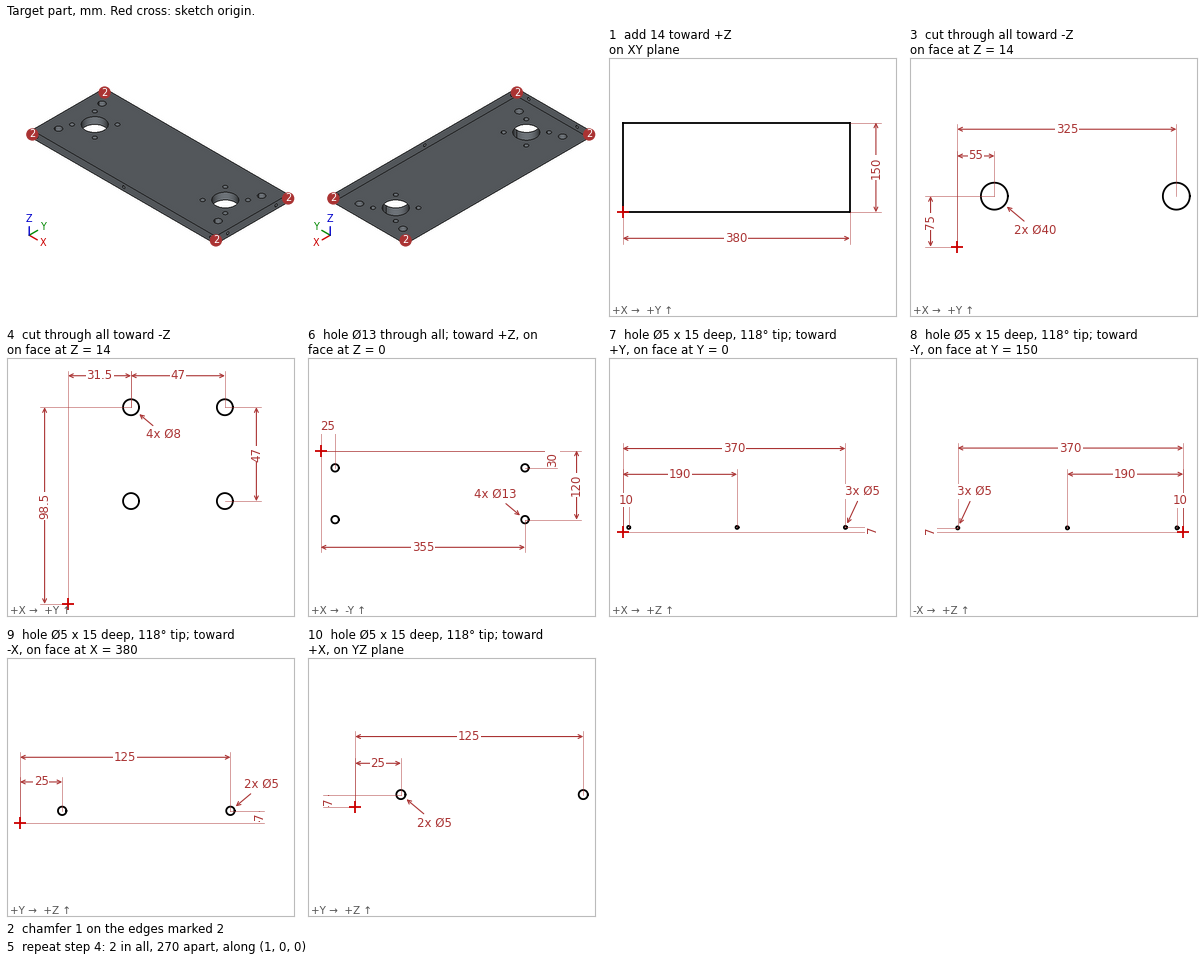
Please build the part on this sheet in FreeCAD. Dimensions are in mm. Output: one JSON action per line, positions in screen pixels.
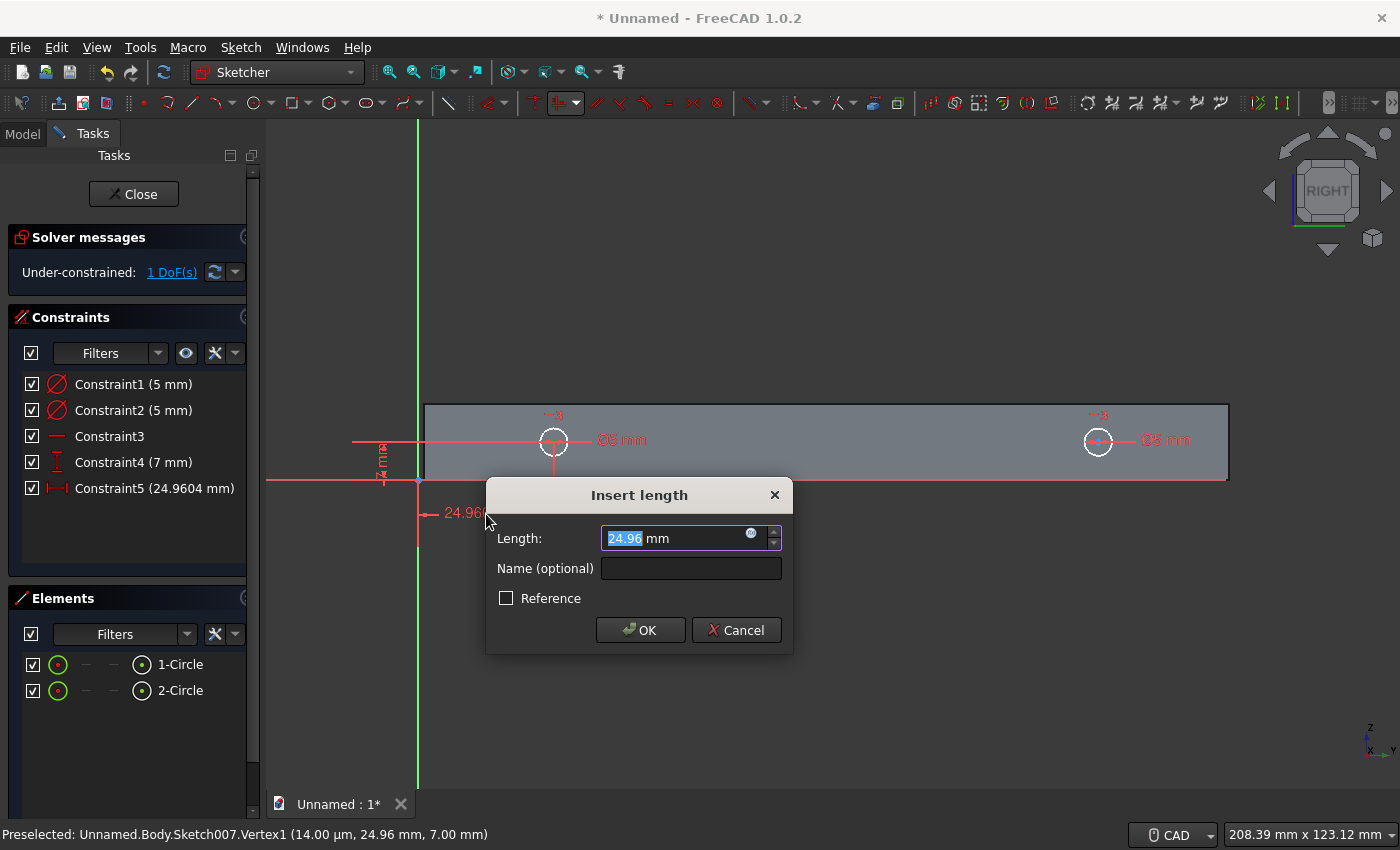
{"action": "type", "text": "25"}
{"action": "key", "text": "Return"}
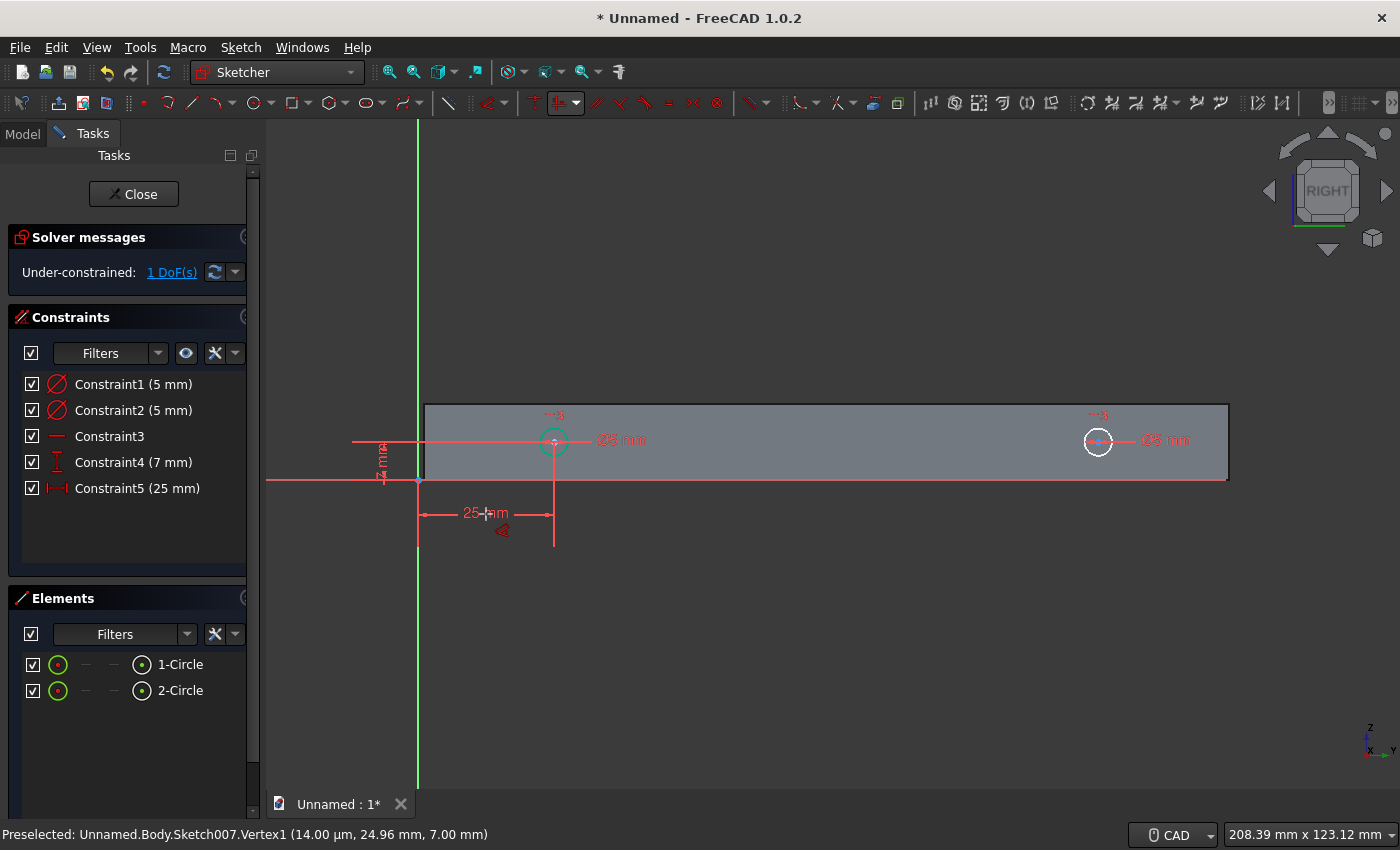
{"action": "left_click", "coordinate": [1098, 442]}
{"action": "left_click", "coordinate": [758, 514]}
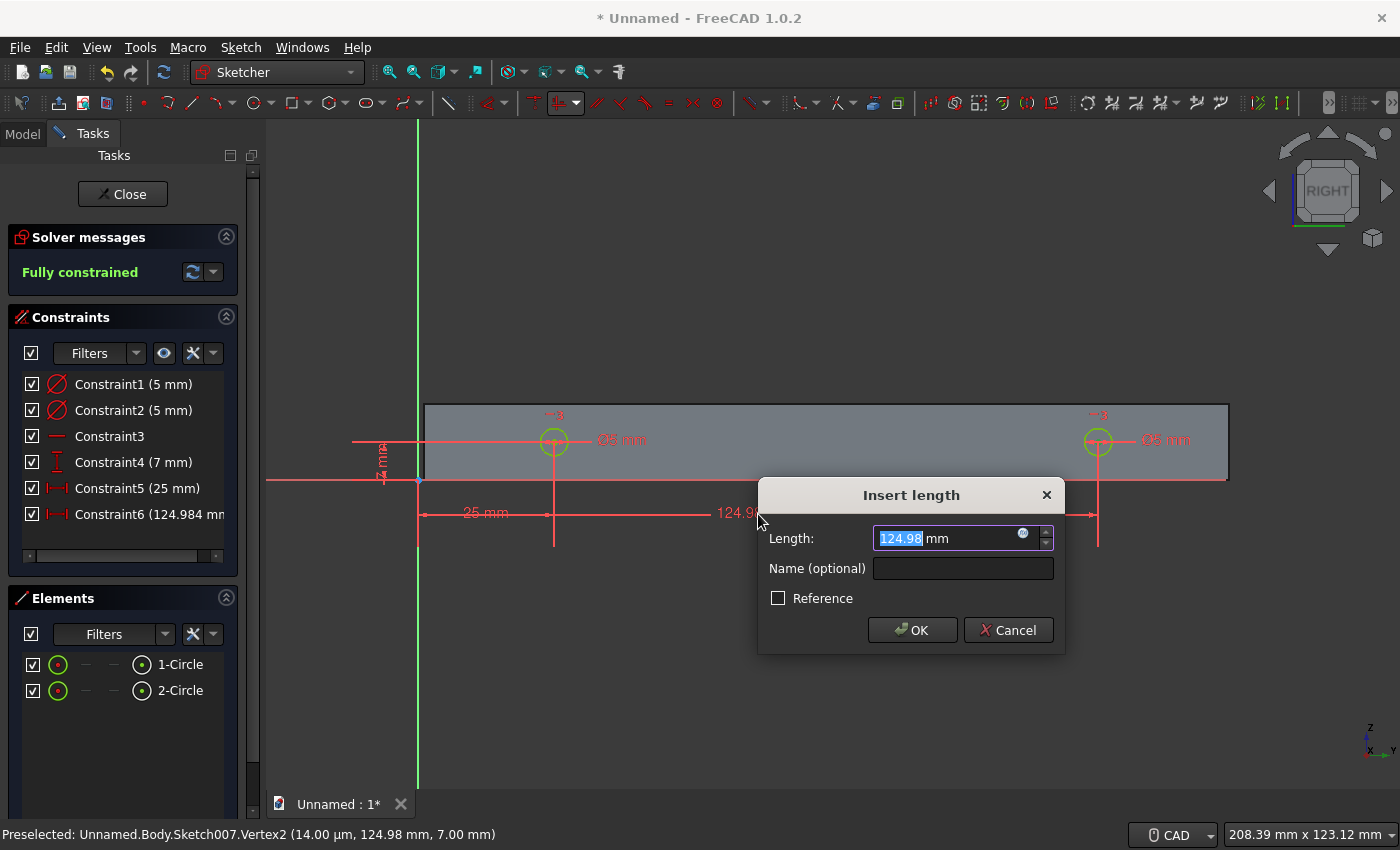
{"action": "type", "text": "125"}
{"action": "key", "text": "Return"}
{"action": "key", "text": "Escape"}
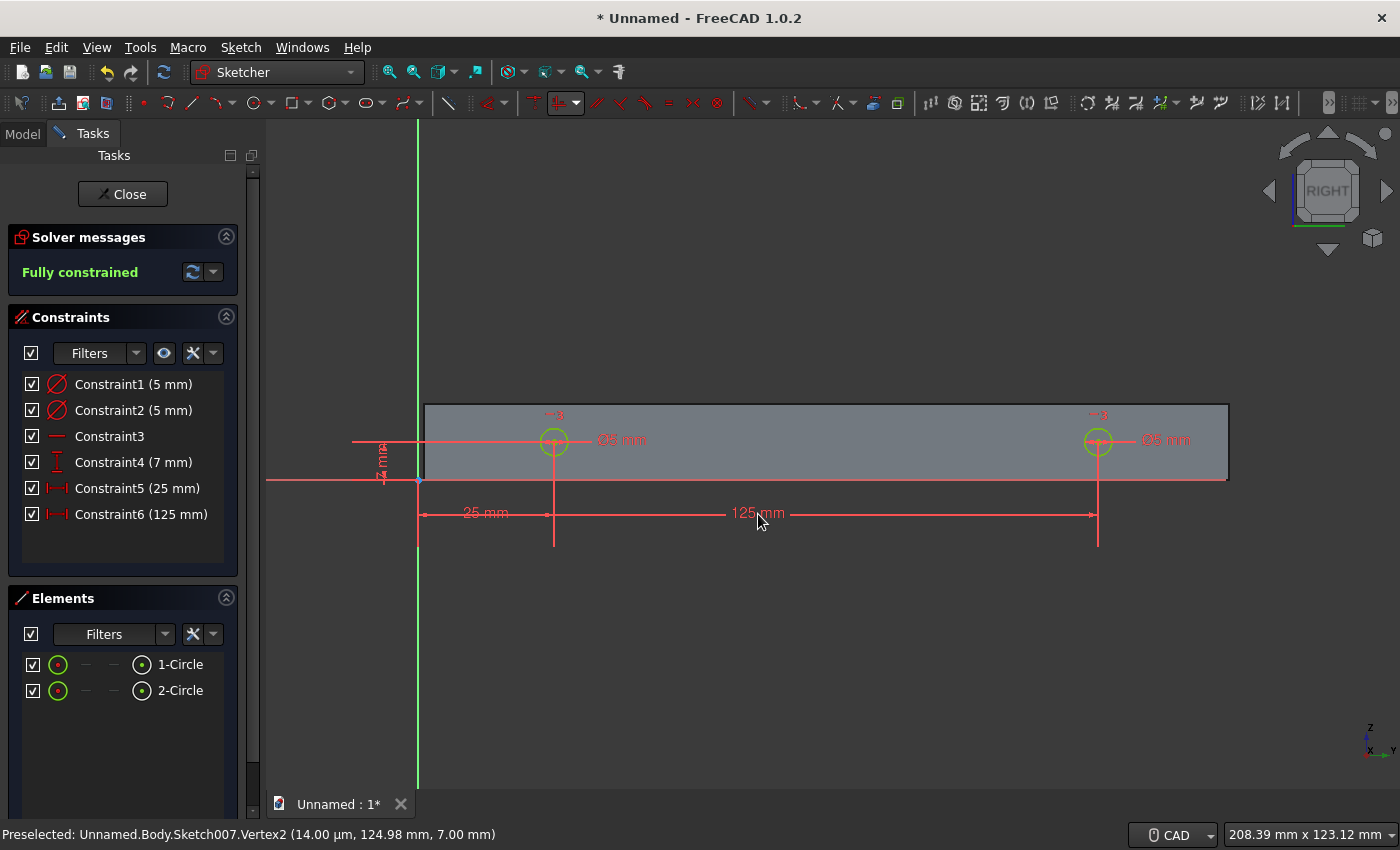
{"action": "left_click", "coordinate": [123, 194]}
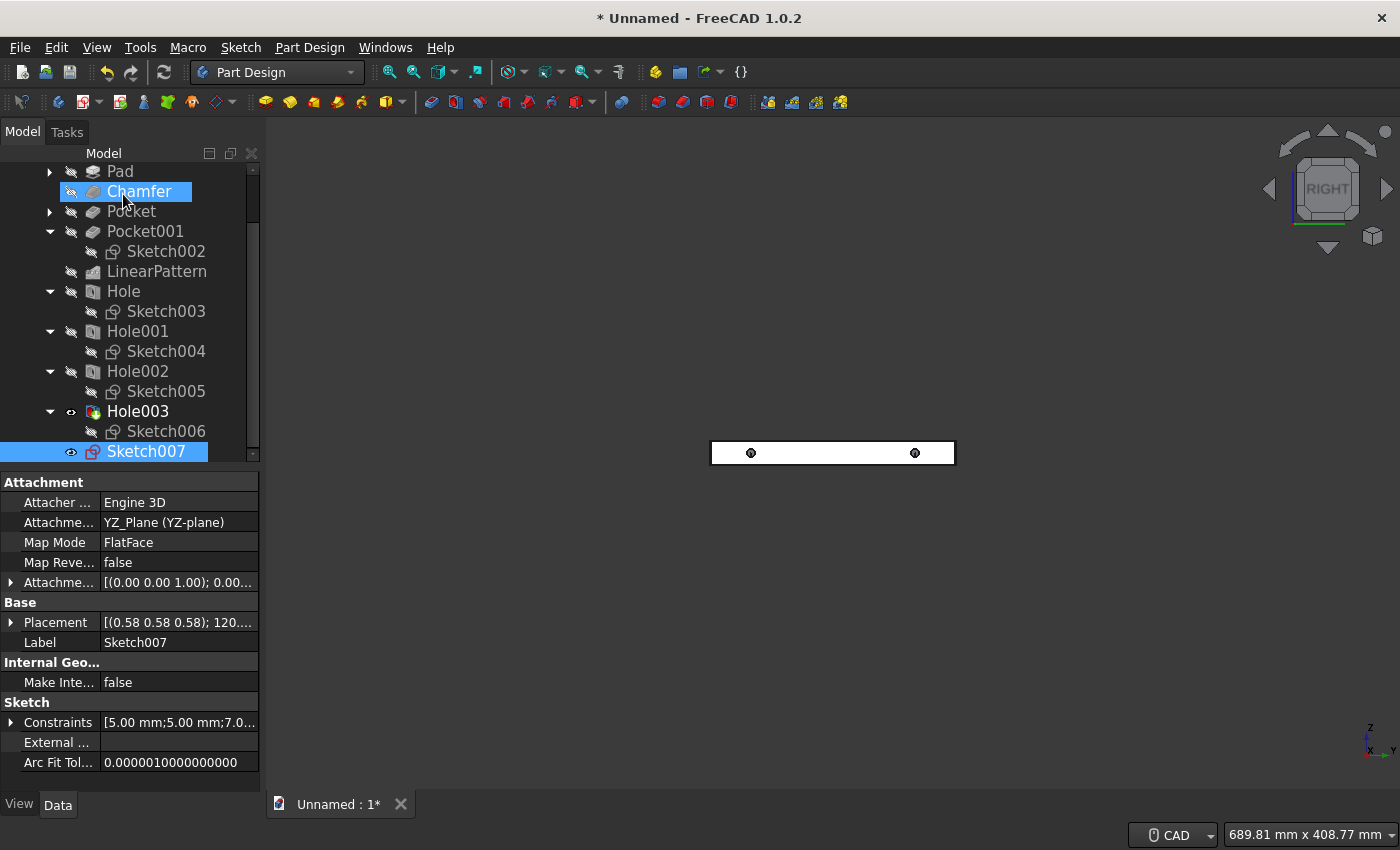
{"action": "left_click", "coordinate": [456, 102]}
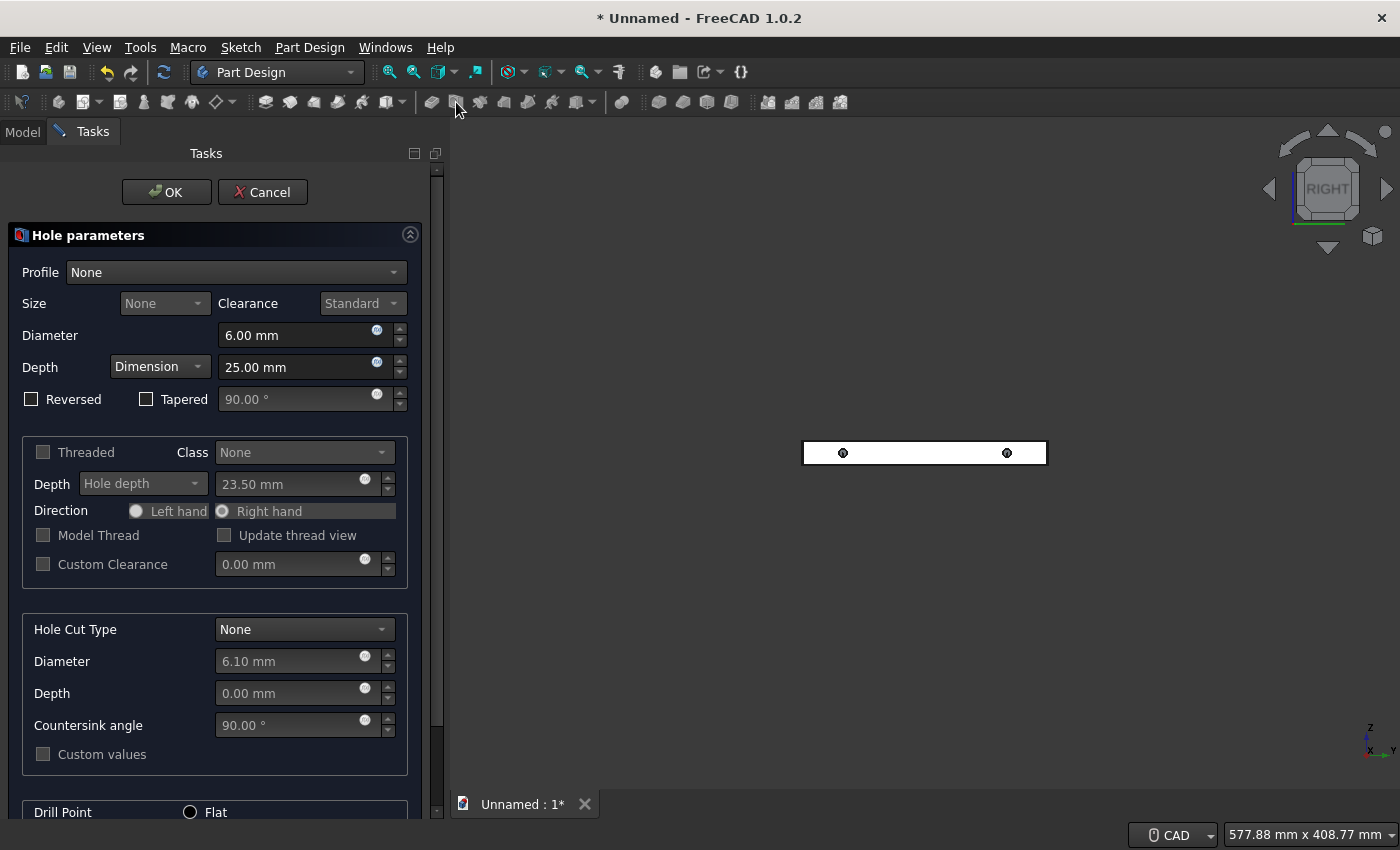
{"action": "triple_click", "coordinate": [305, 335]}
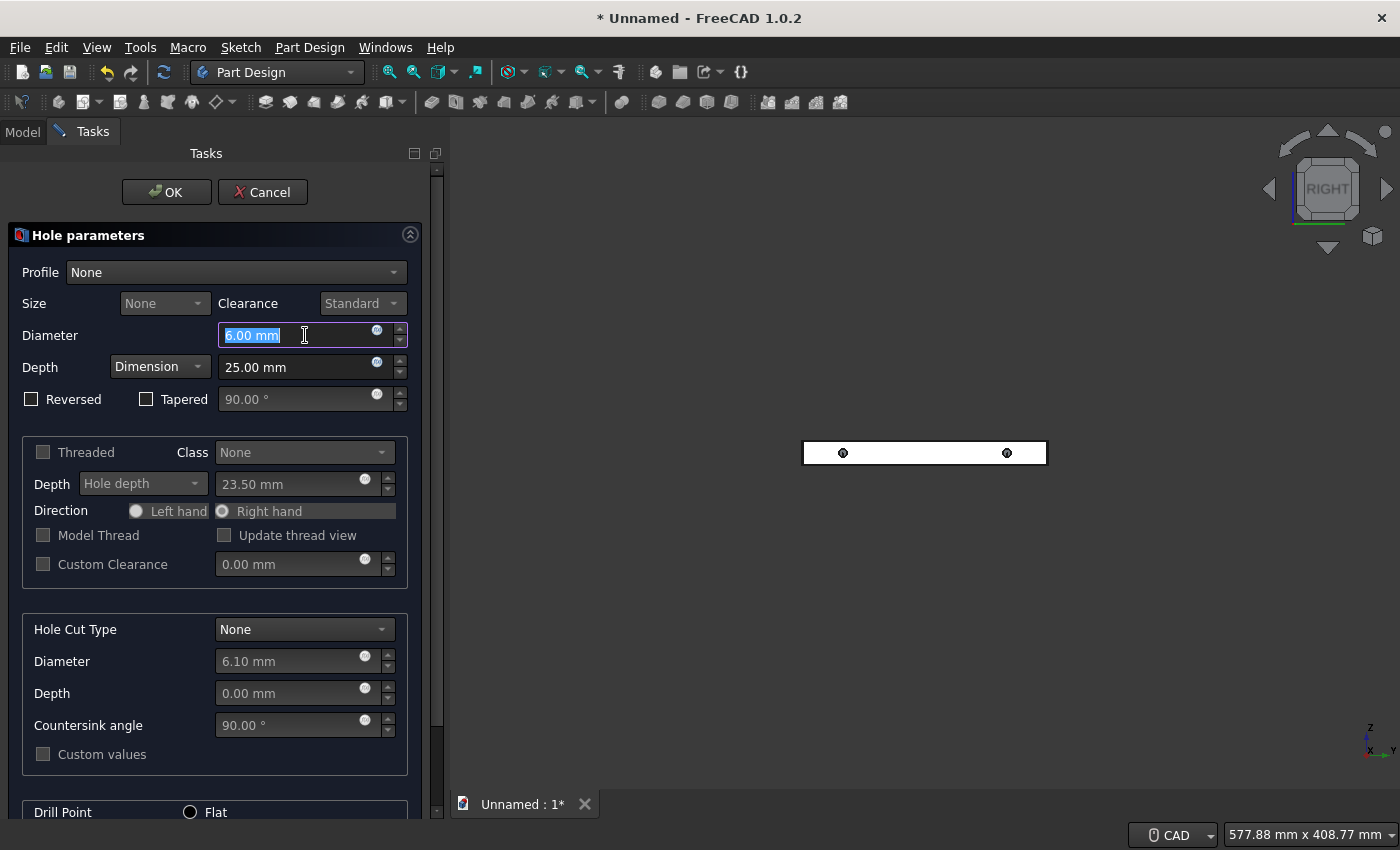
{"action": "type", "text": "5"}
{"action": "key", "text": "Tab"}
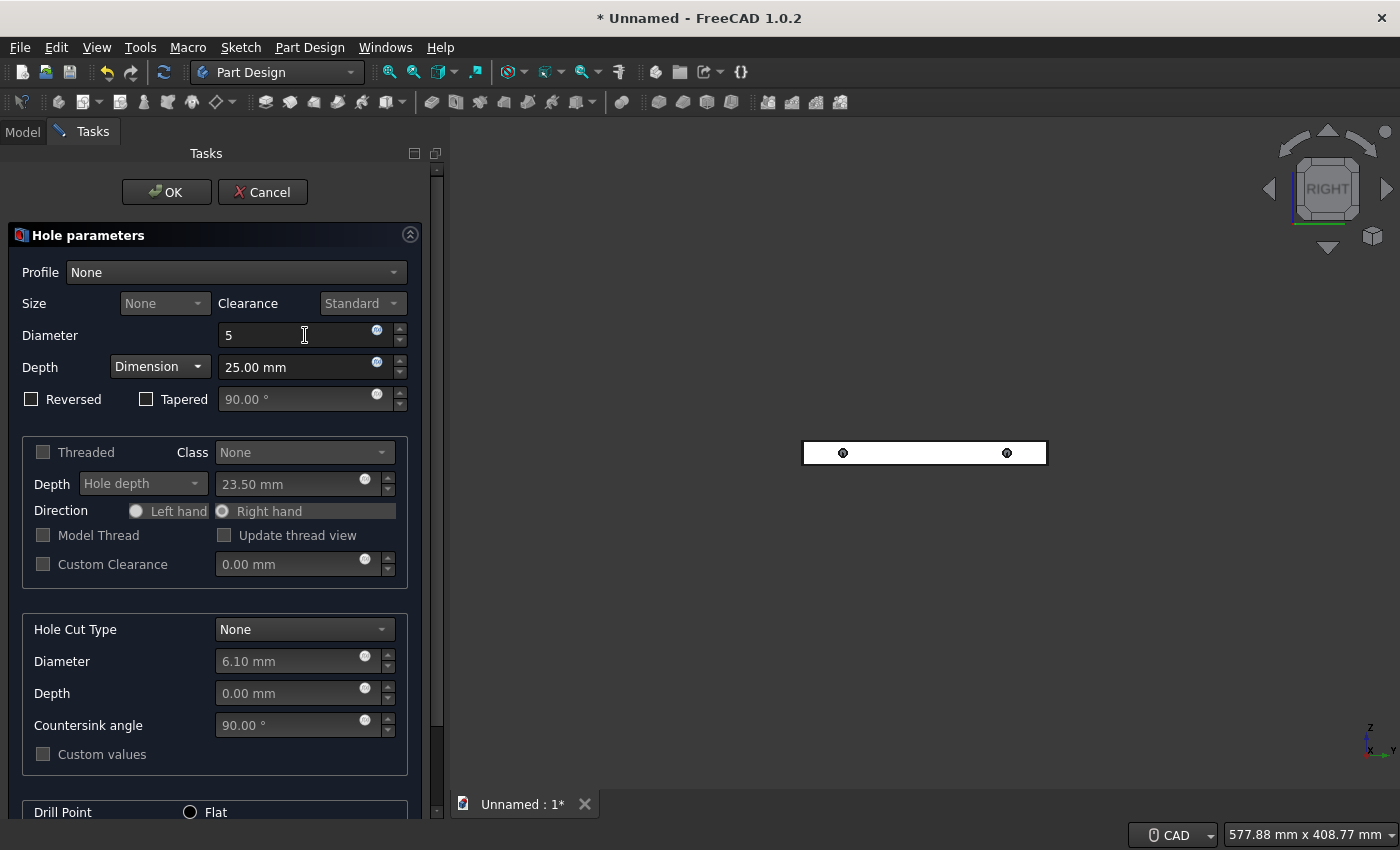
{"action": "triple_click", "coordinate": [305, 367]}